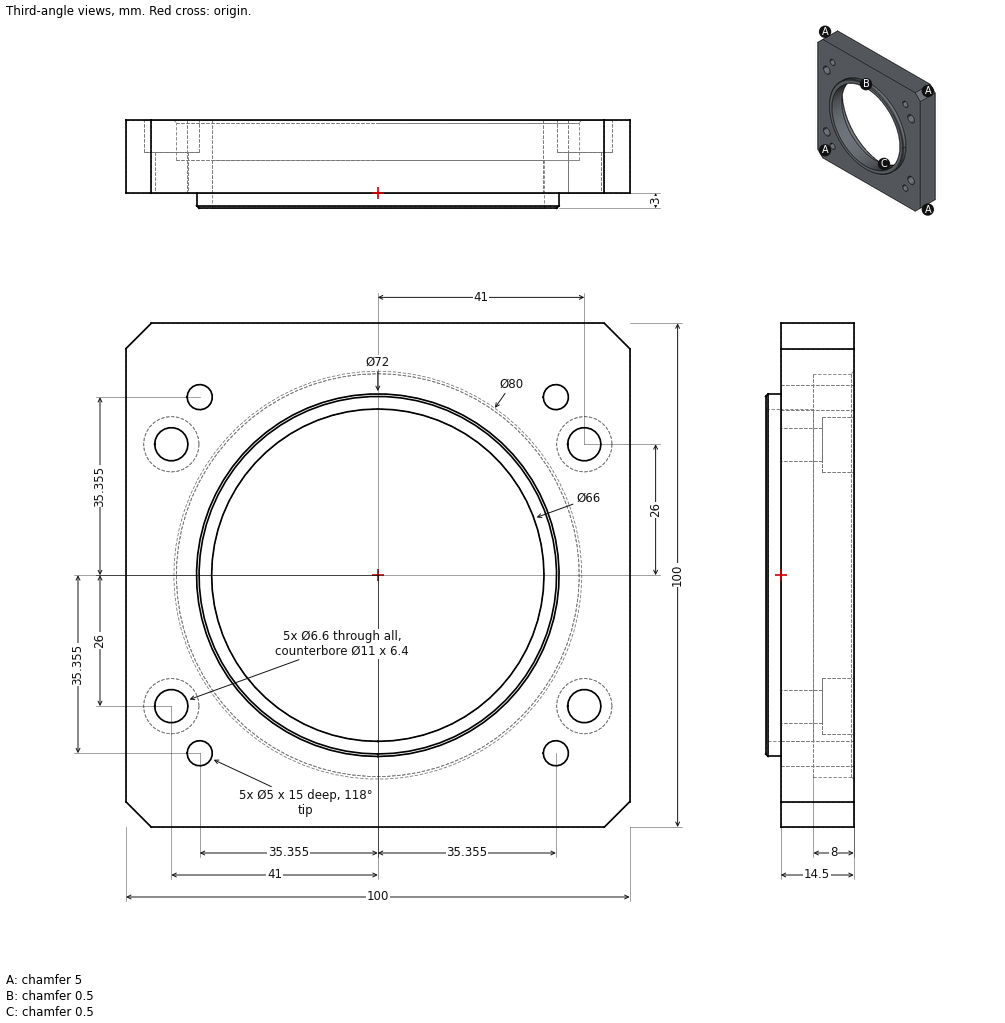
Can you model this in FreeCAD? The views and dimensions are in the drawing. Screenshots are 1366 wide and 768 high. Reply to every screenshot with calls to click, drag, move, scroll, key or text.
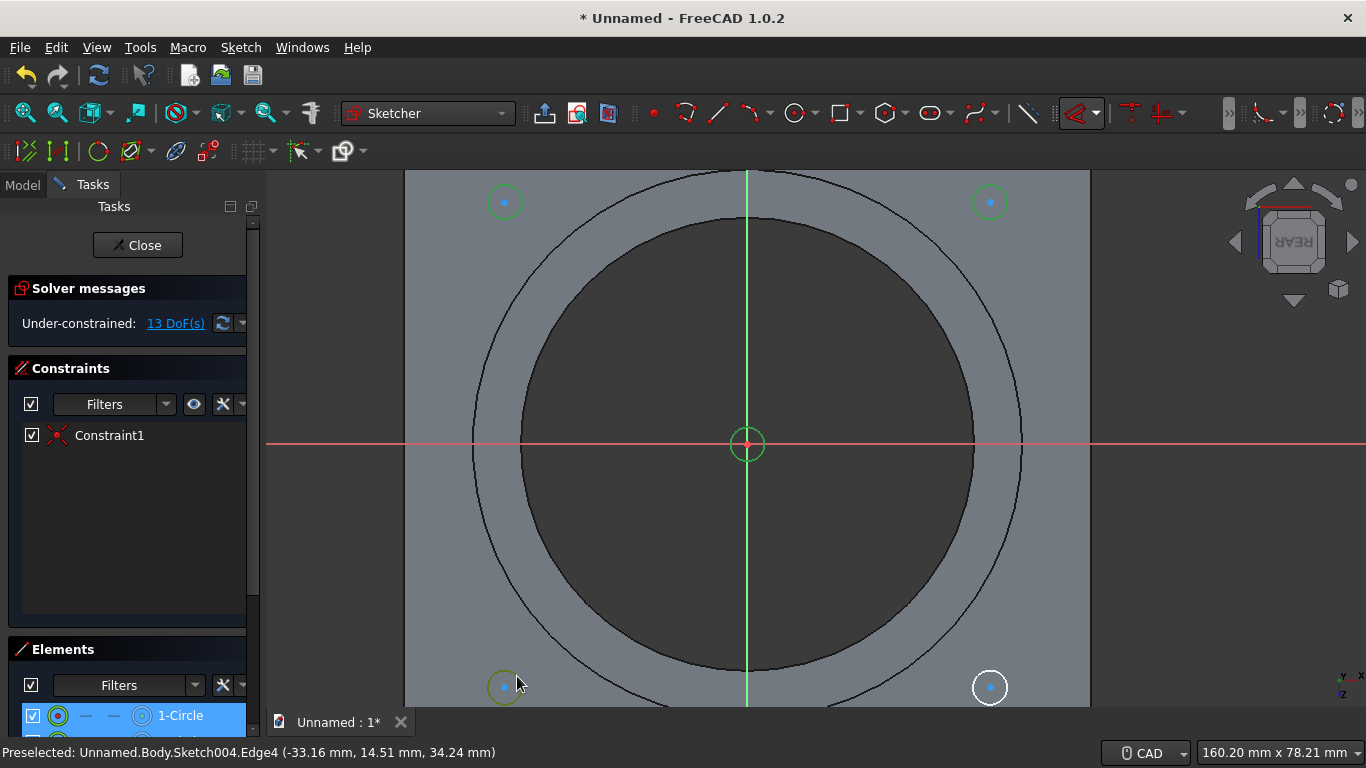
click(1002, 676)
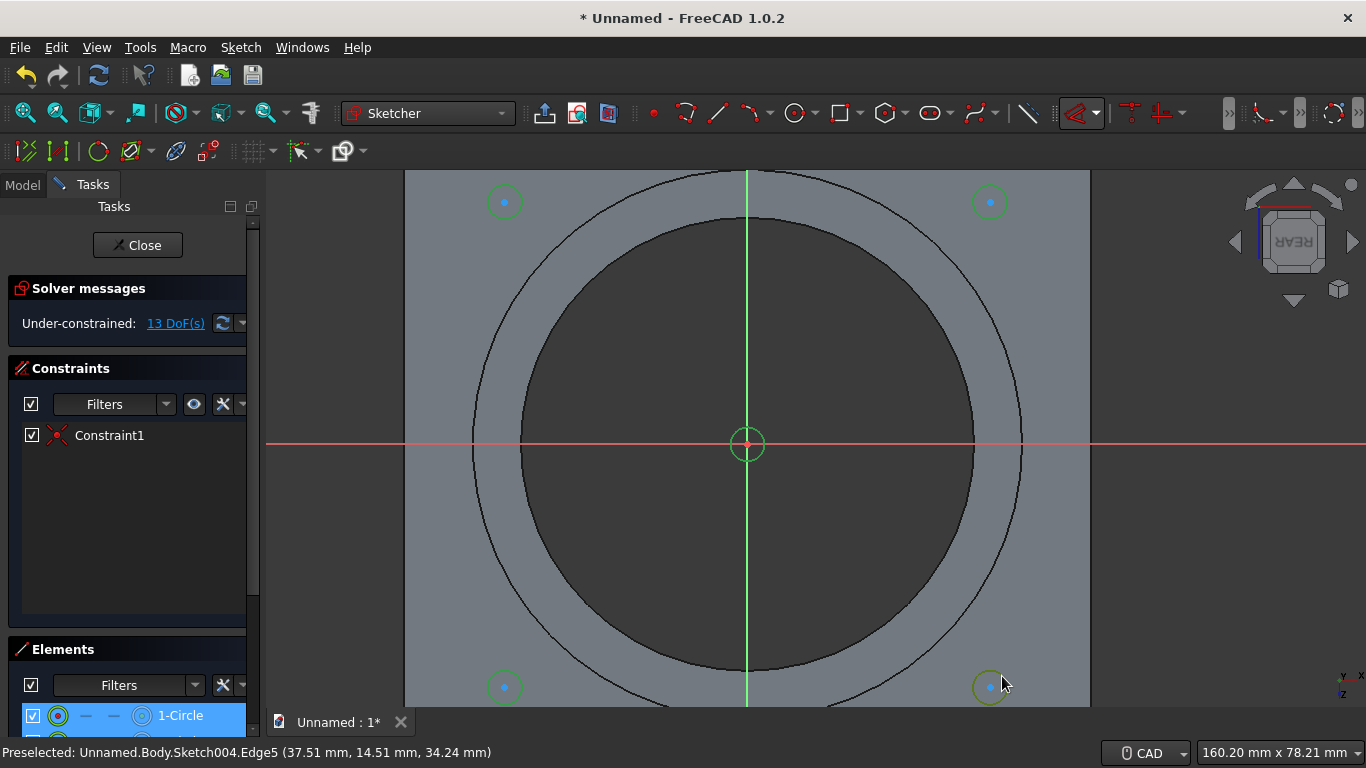
key(e)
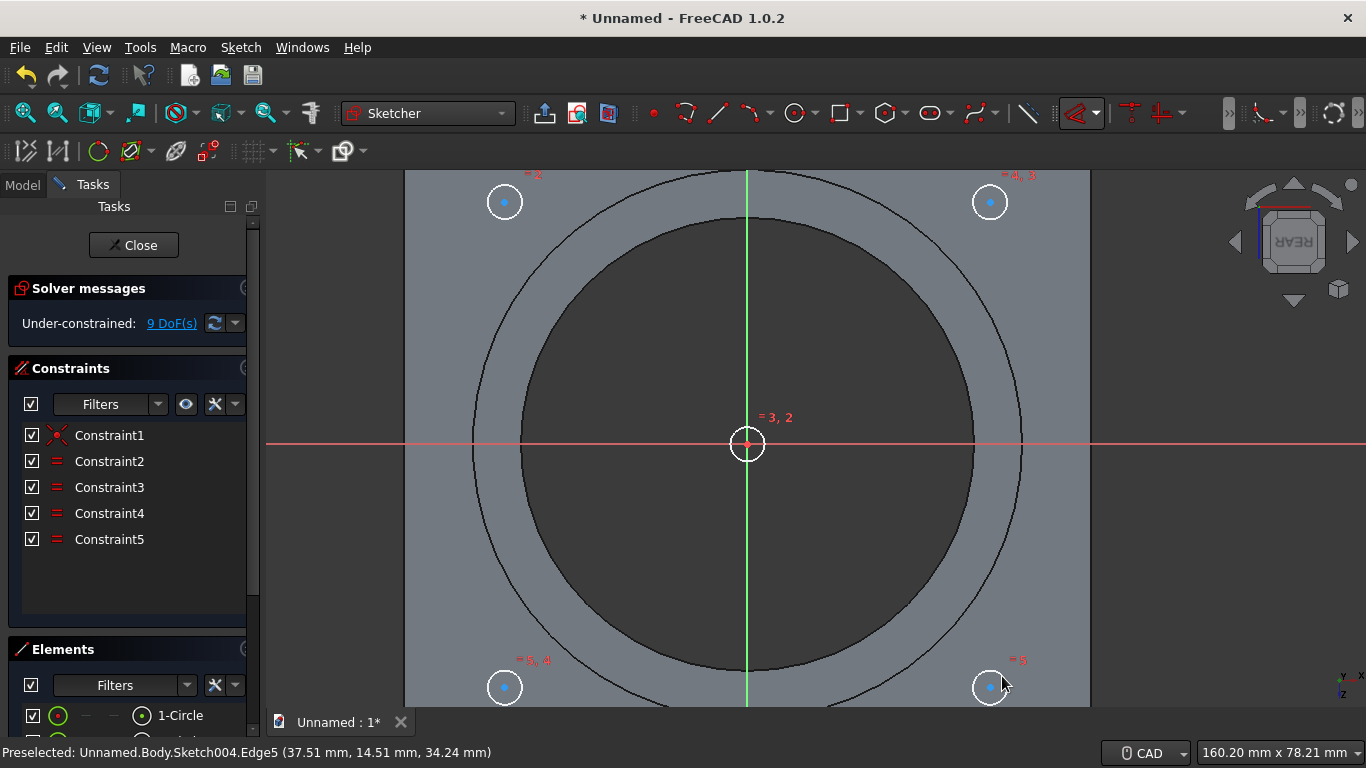
click(505, 202)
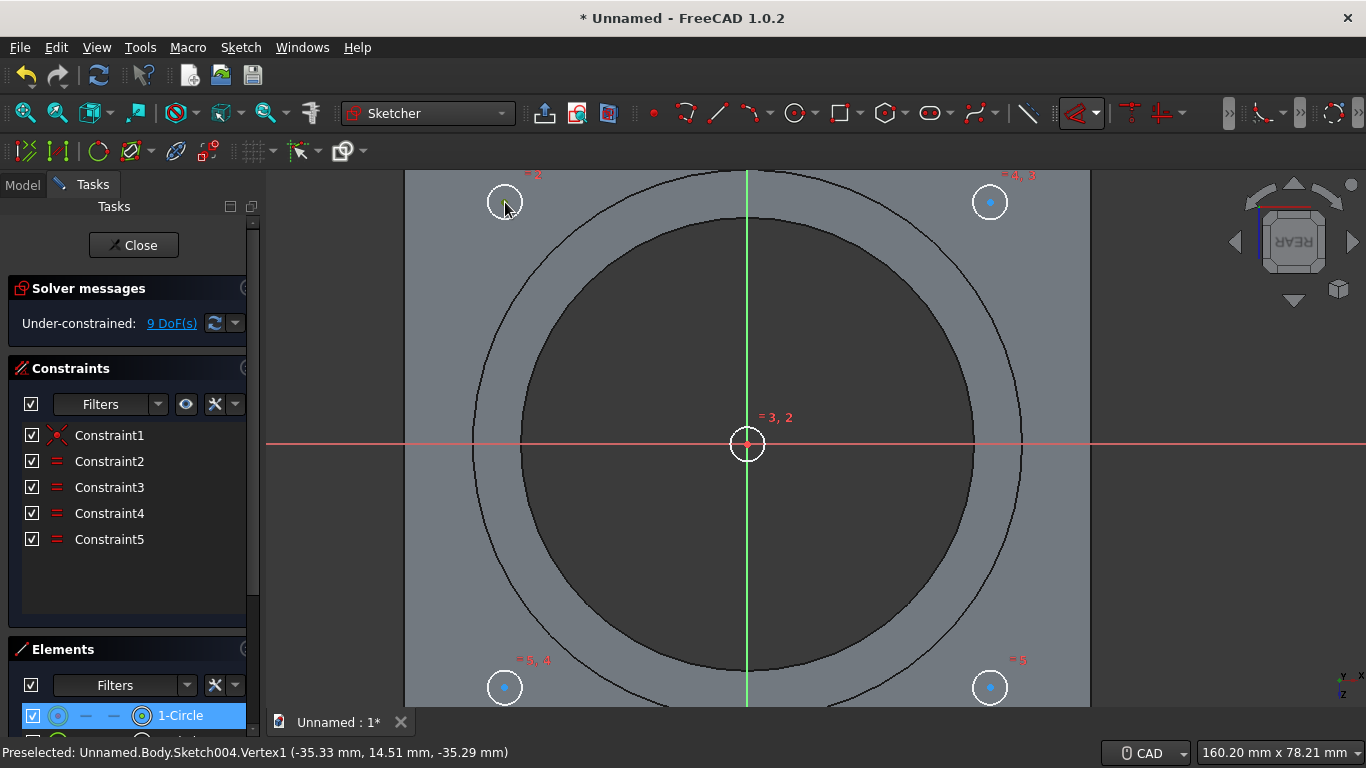
click(990, 202)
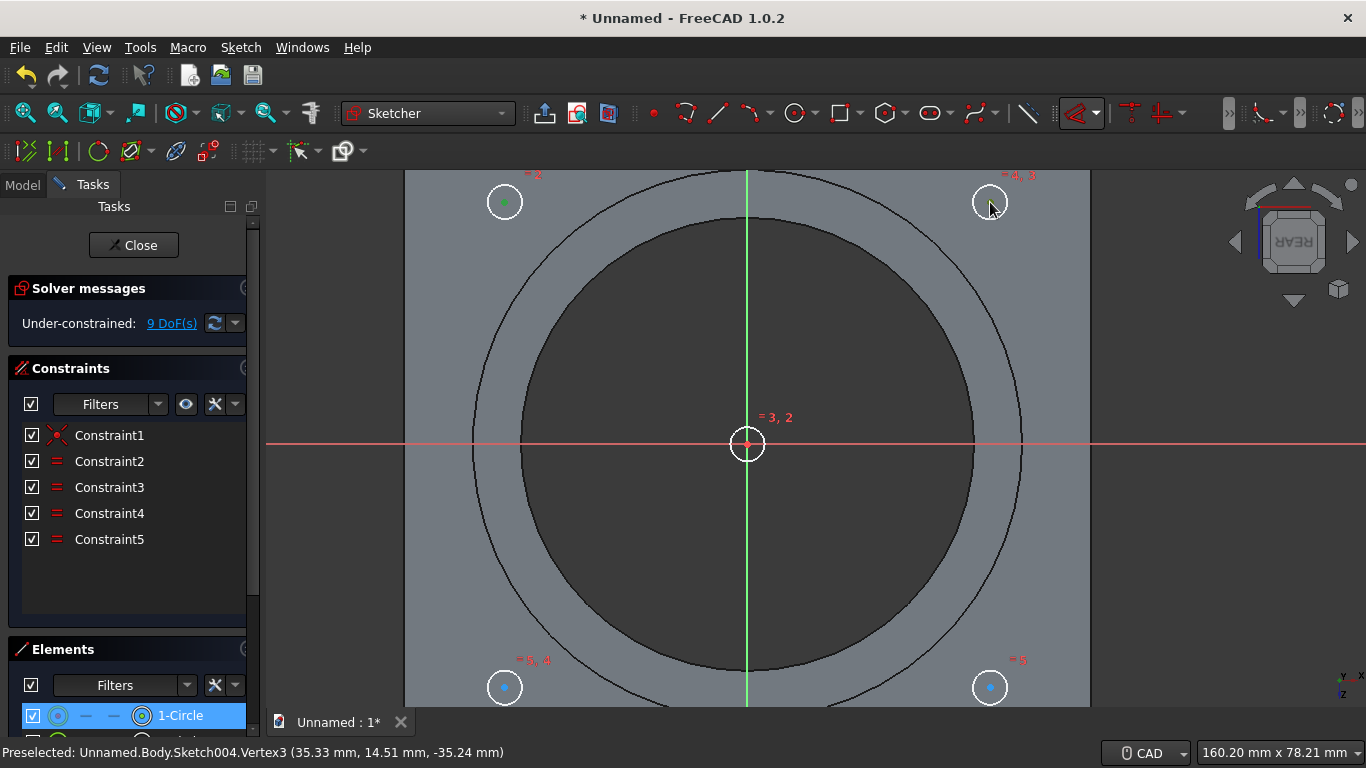
click(1184, 114)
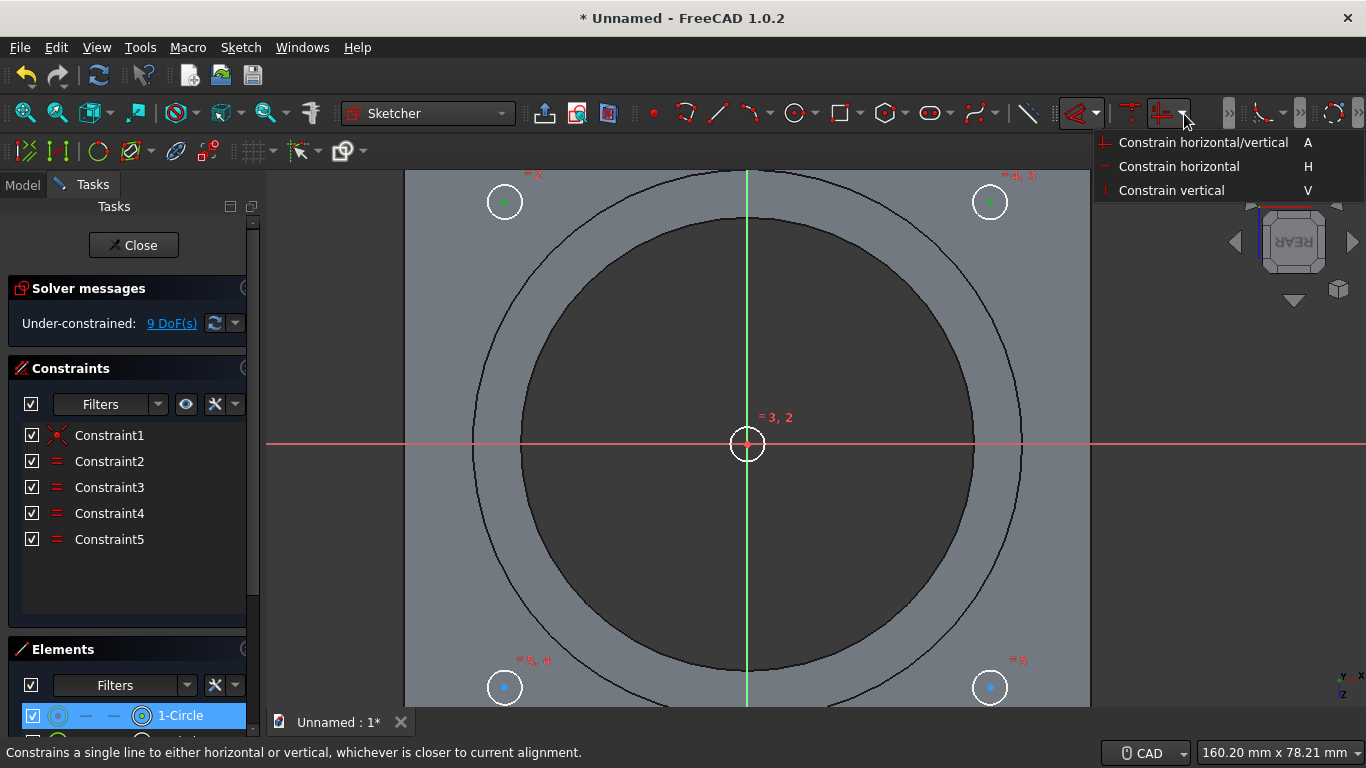
click(1229, 166)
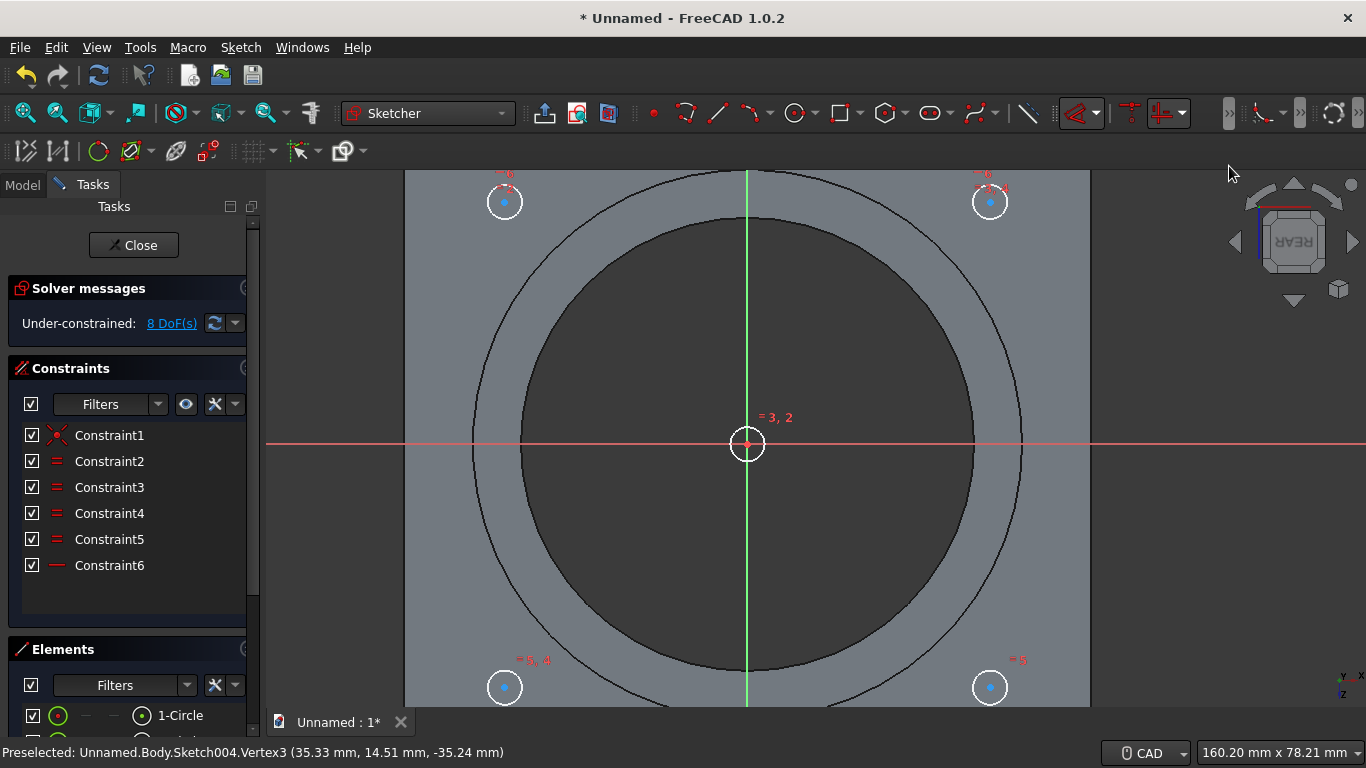
click(505, 202)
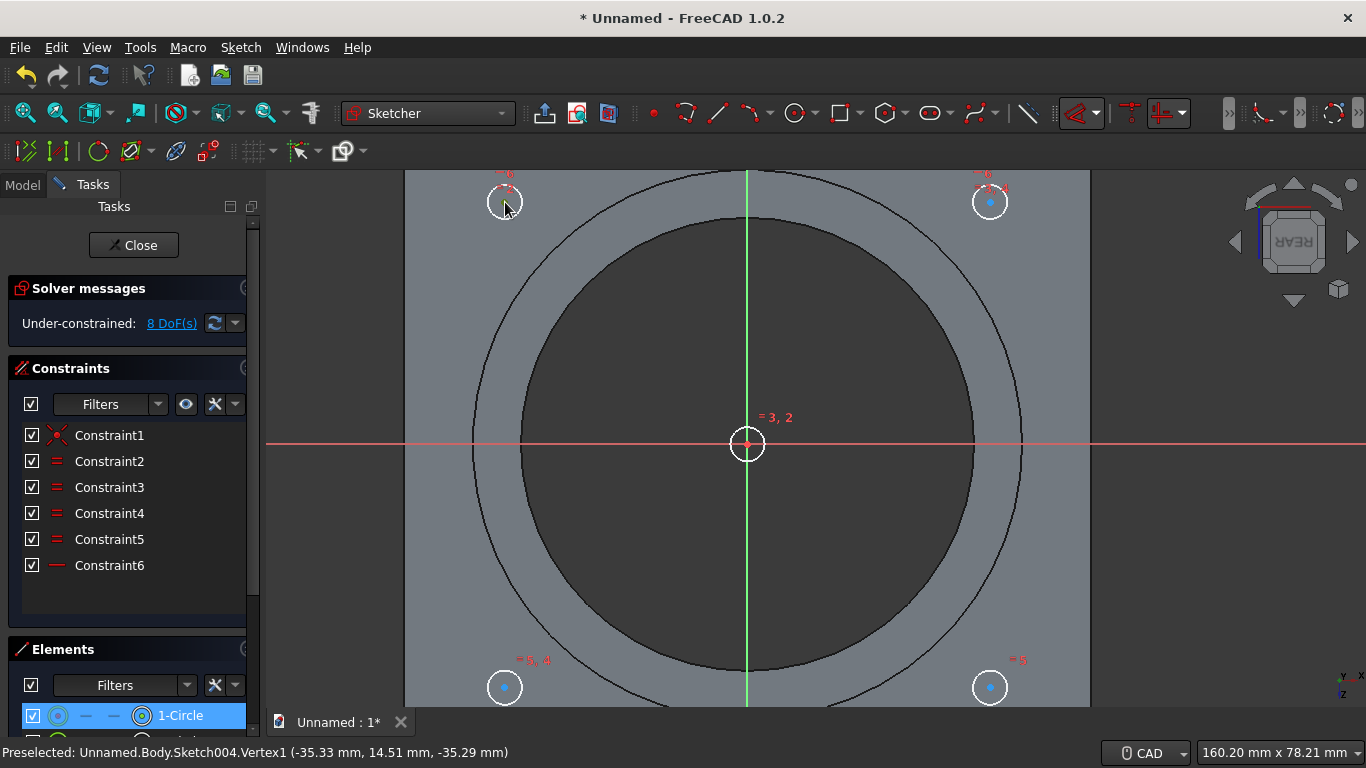
scroll(748, 427, down, 2)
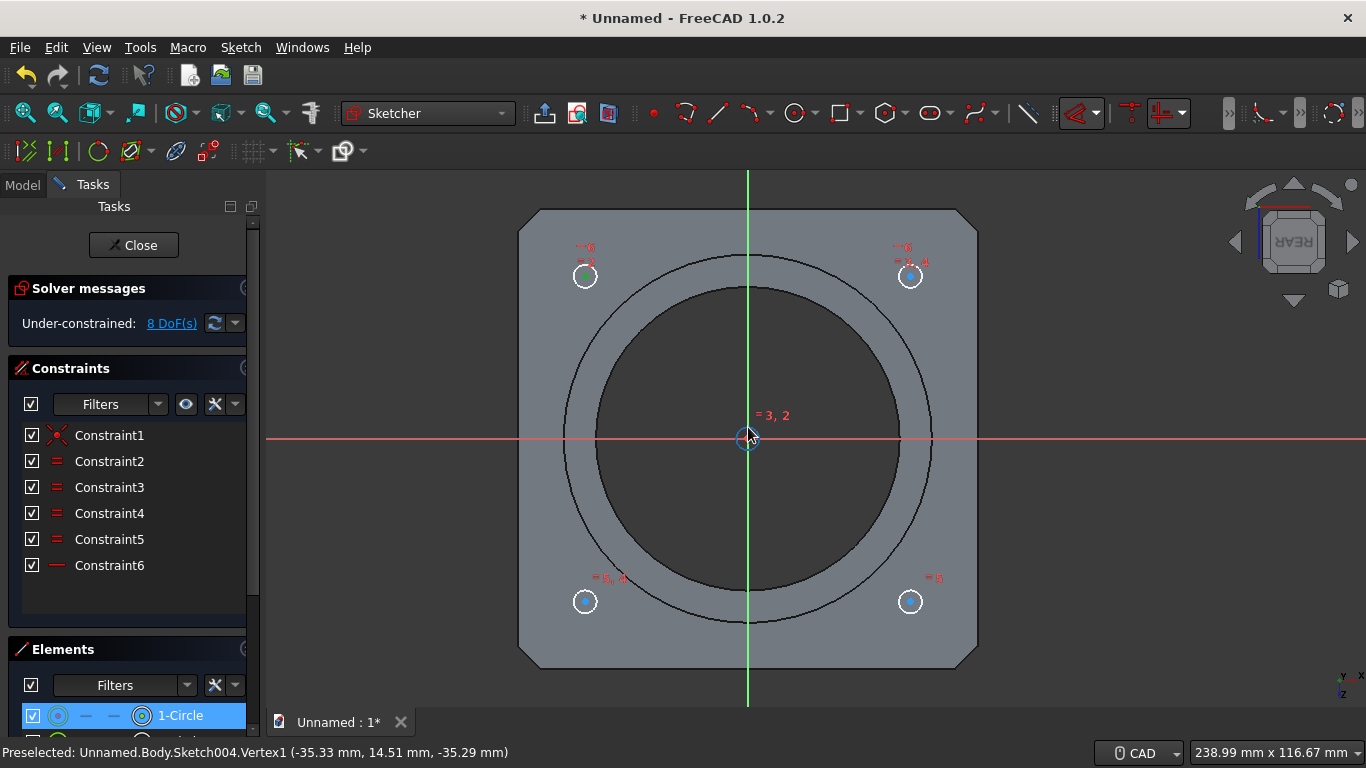
click(585, 602)